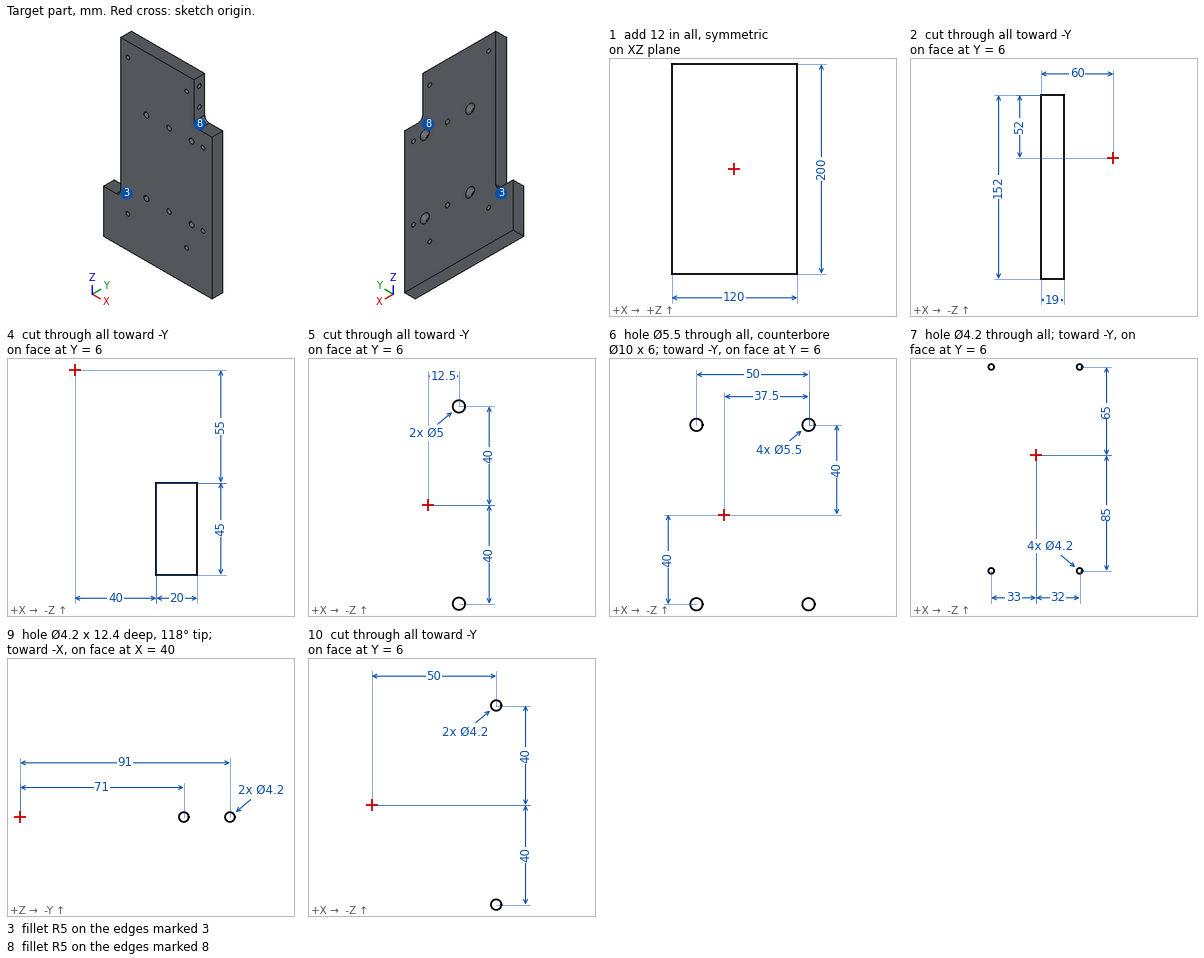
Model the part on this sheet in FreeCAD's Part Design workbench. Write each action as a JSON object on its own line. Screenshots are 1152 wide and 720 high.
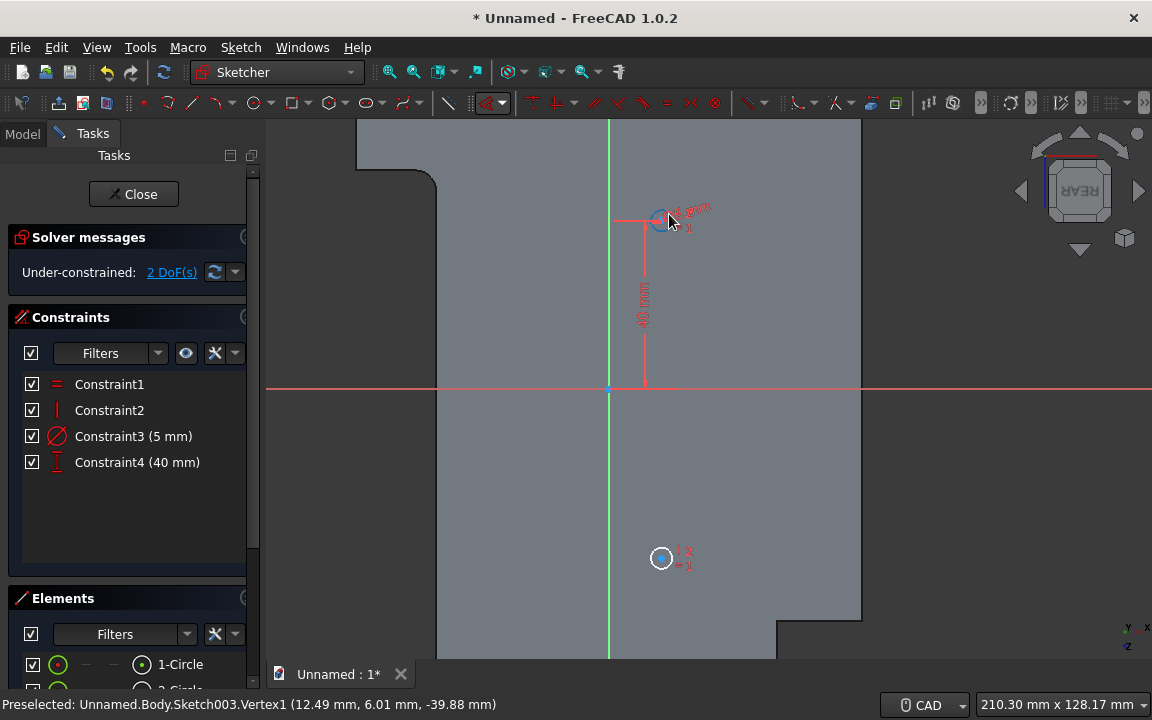
{"action": "left_click", "coordinate": [662, 558]}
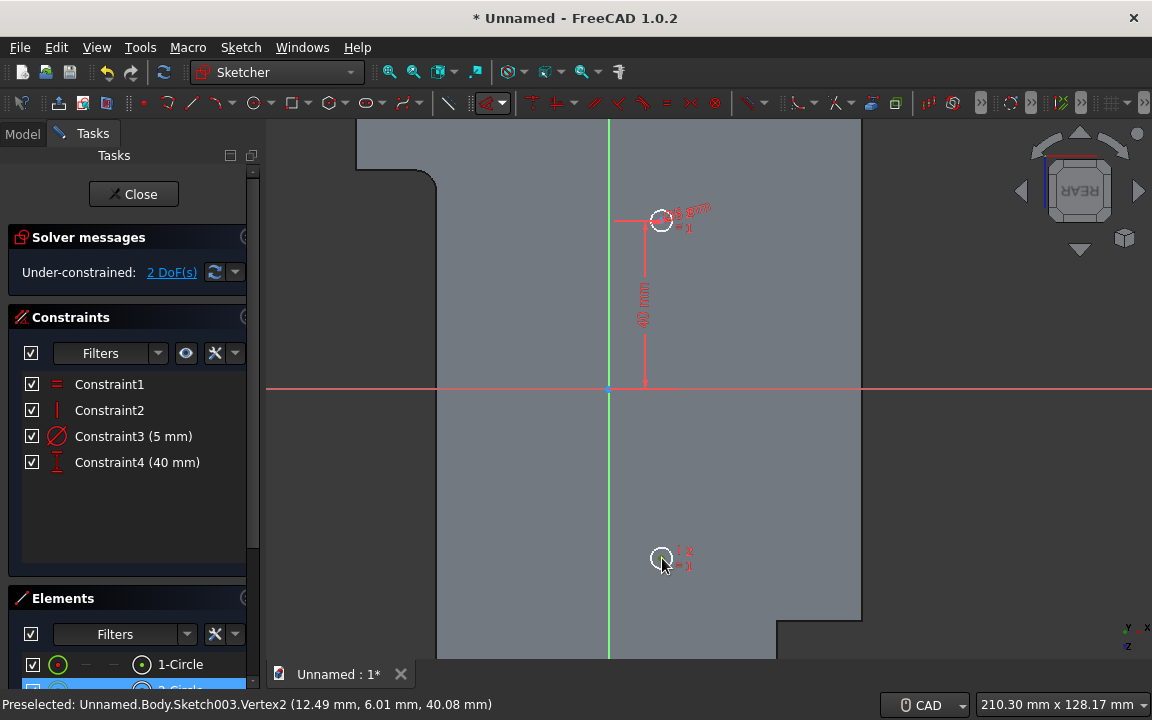
{"action": "left_click", "coordinate": [504, 104]}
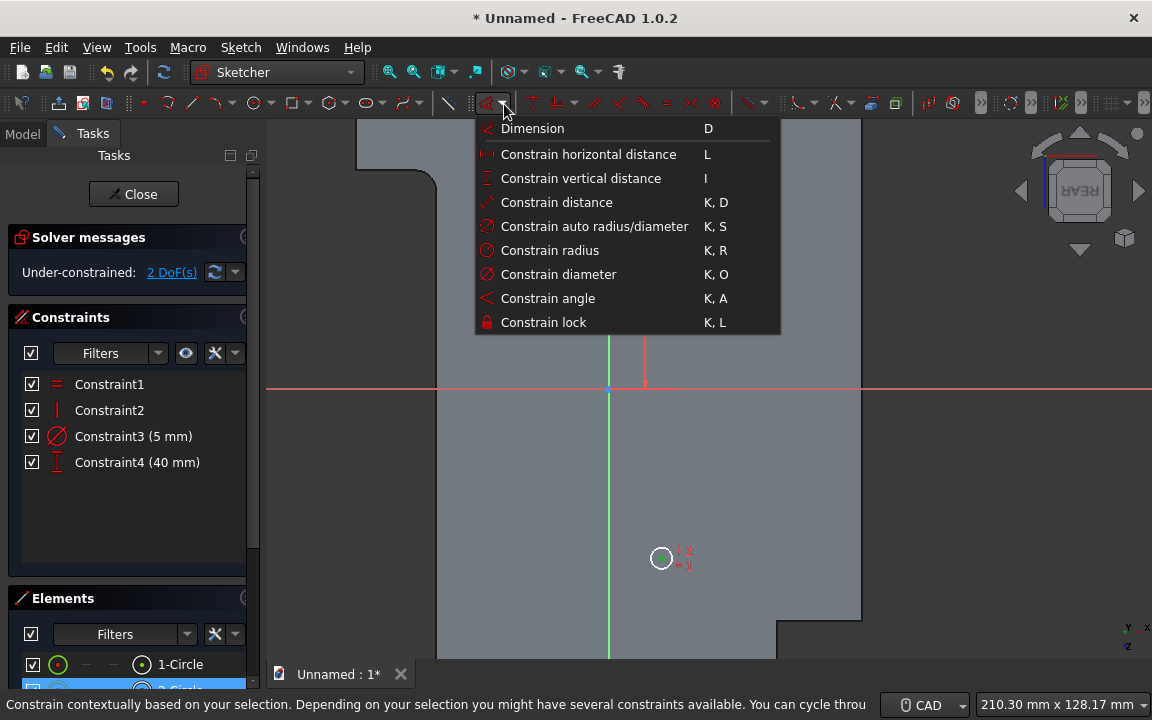
{"action": "left_click", "coordinate": [628, 178]}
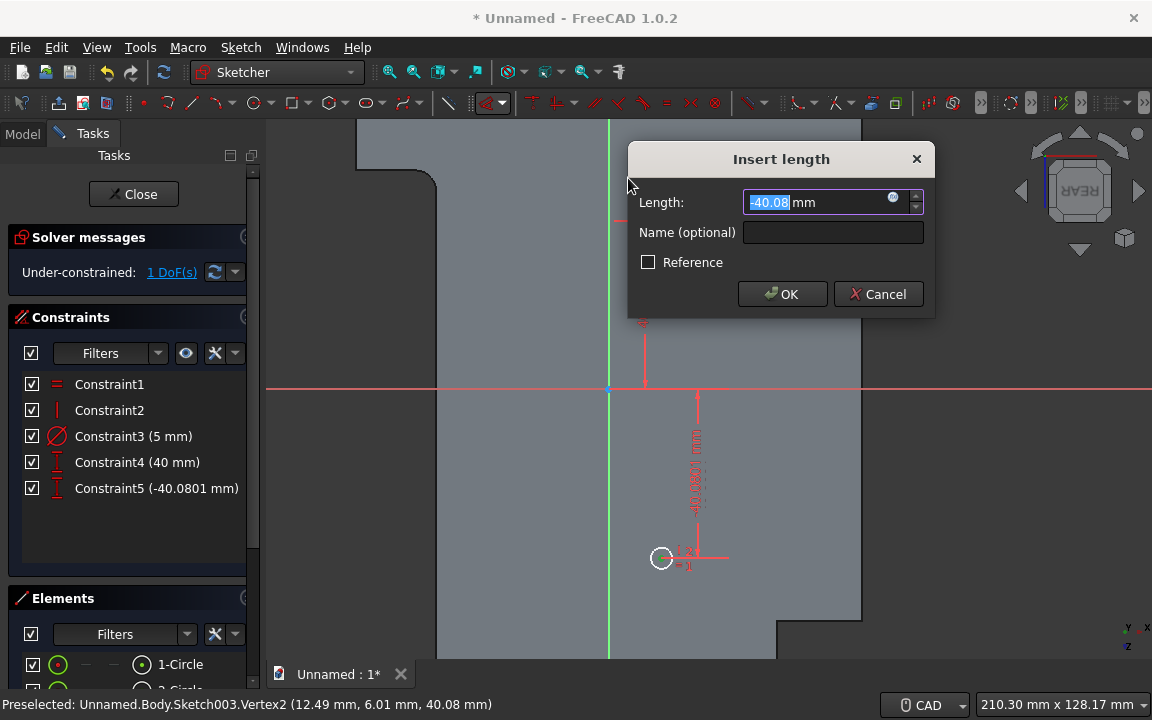
{"action": "type", "text": "-40"}
{"action": "key", "text": "Return"}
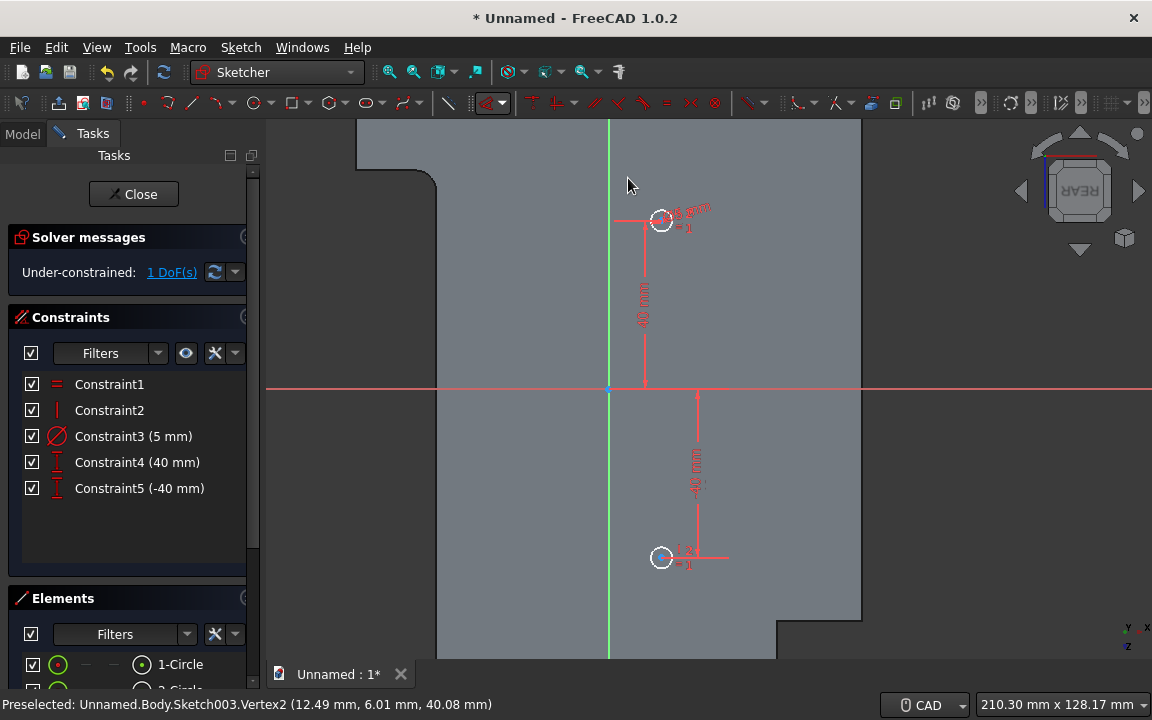
{"action": "left_click", "coordinate": [662, 221]}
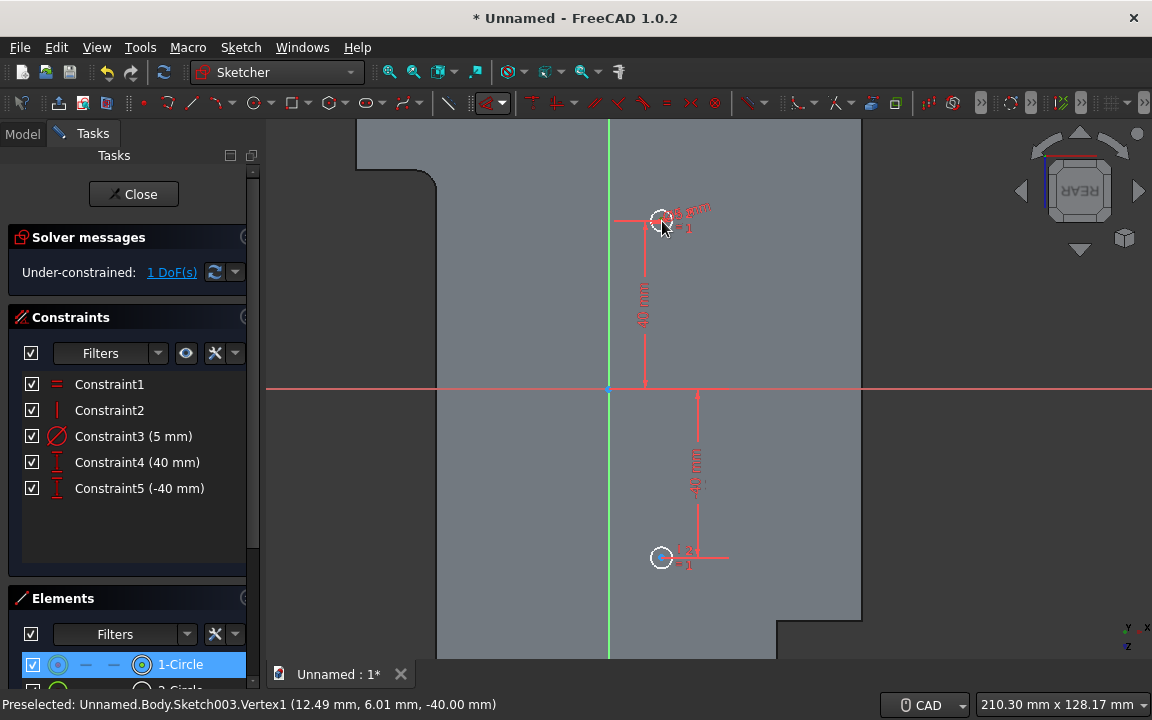
{"action": "key", "text": "l"}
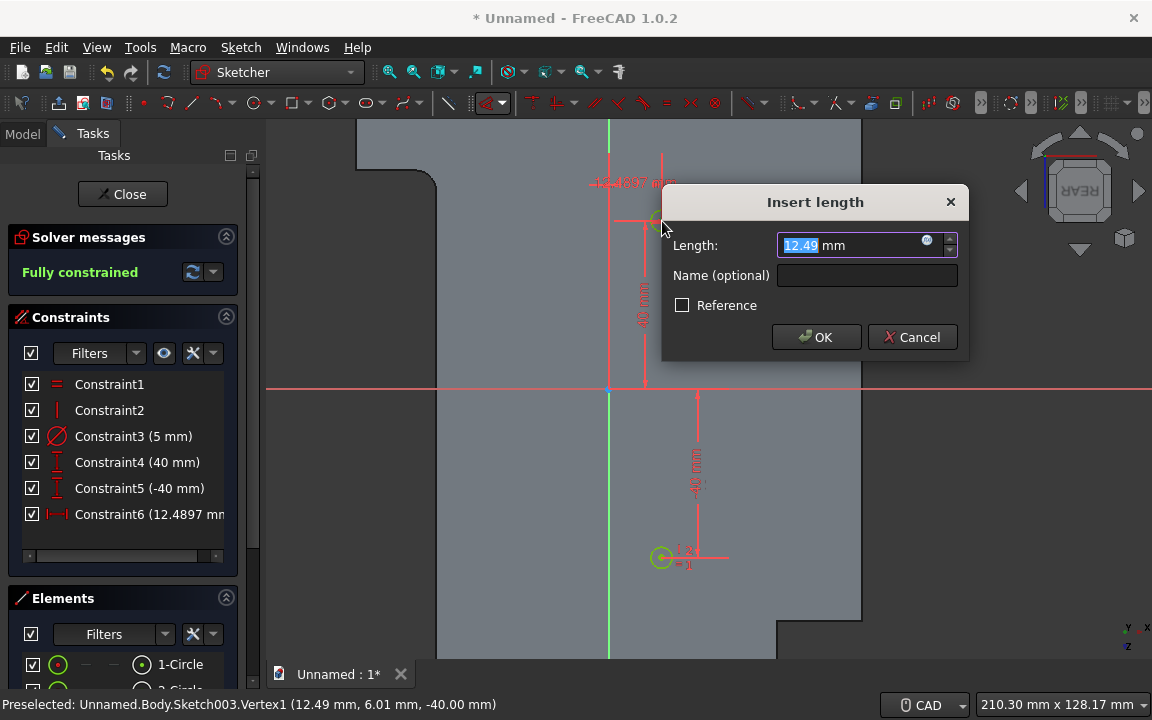
{"action": "type", "text": "12.5"}
{"action": "key", "text": "Return"}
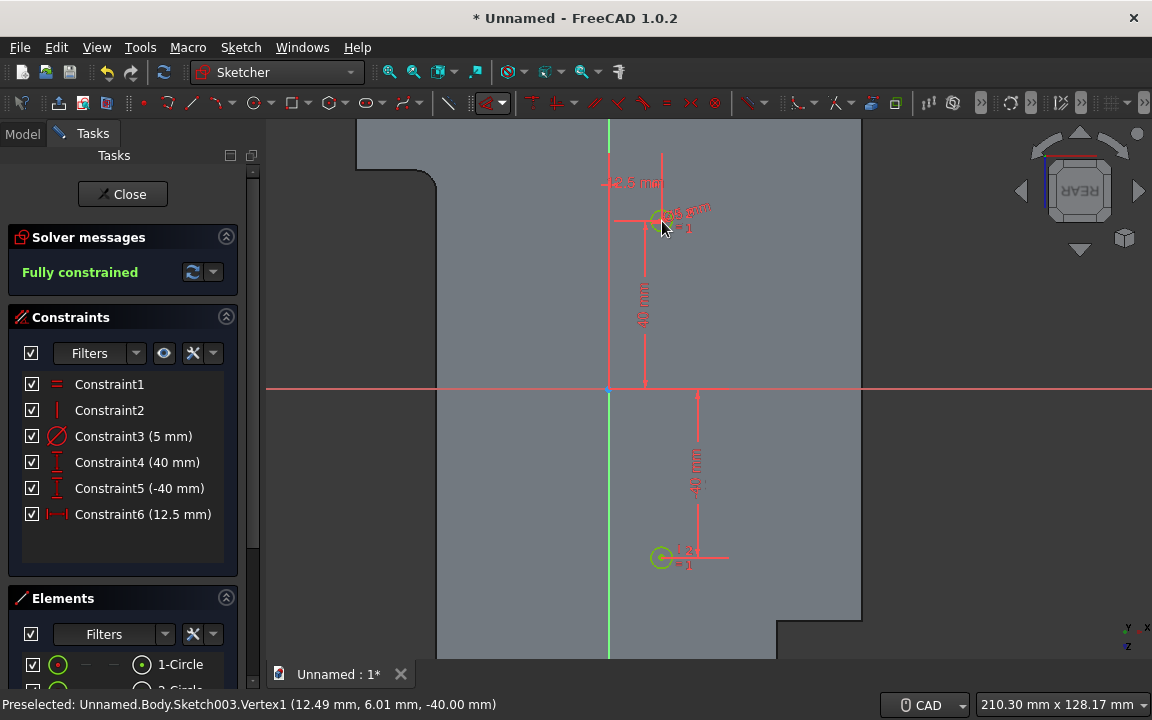
{"action": "left_click", "coordinate": [123, 194]}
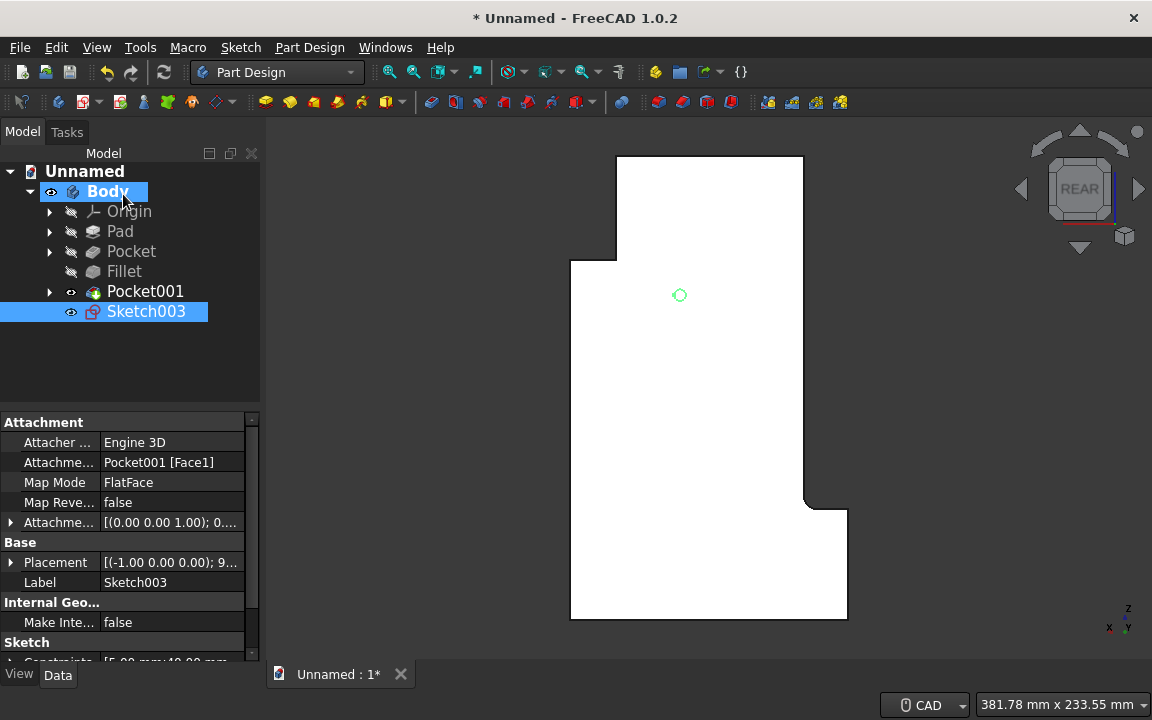
{"action": "left_click", "coordinate": [432, 102]}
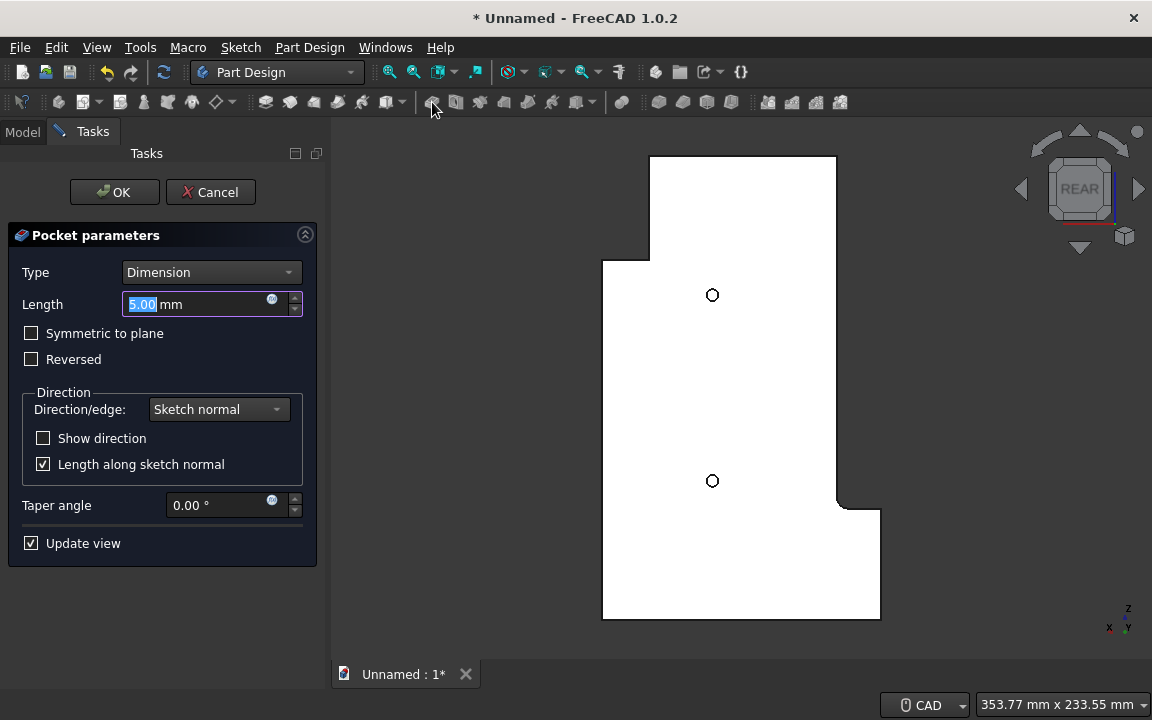
{"action": "left_click", "coordinate": [212, 272]}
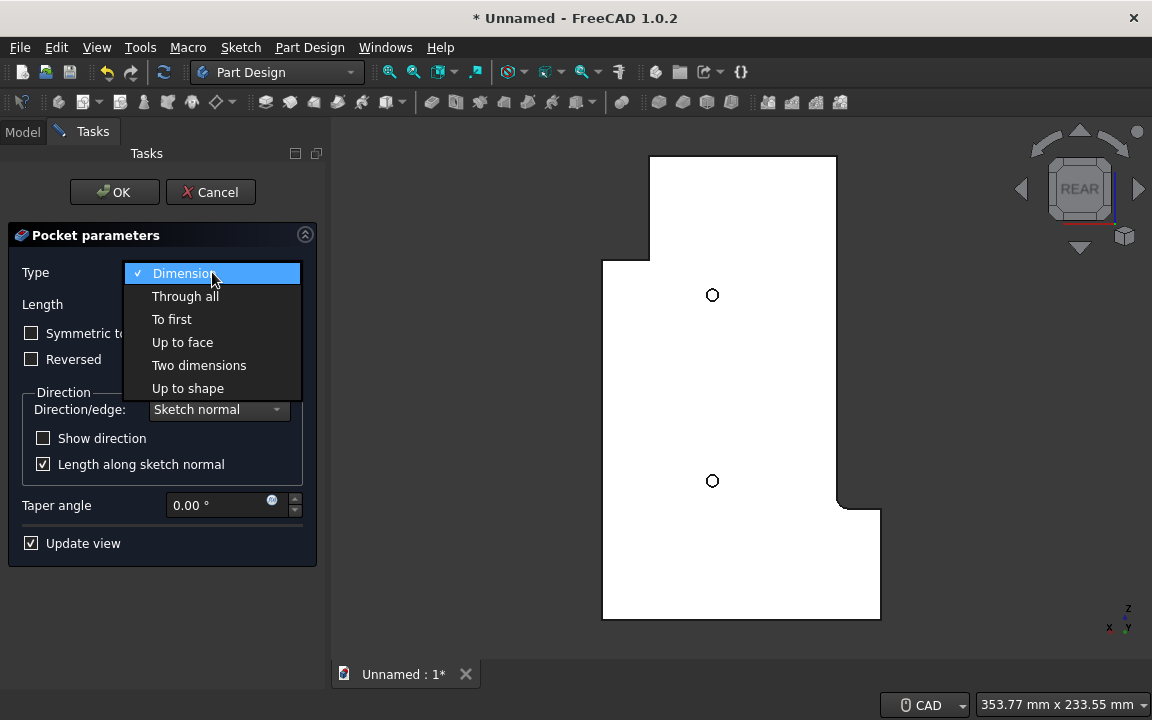
{"action": "left_click", "coordinate": [212, 296]}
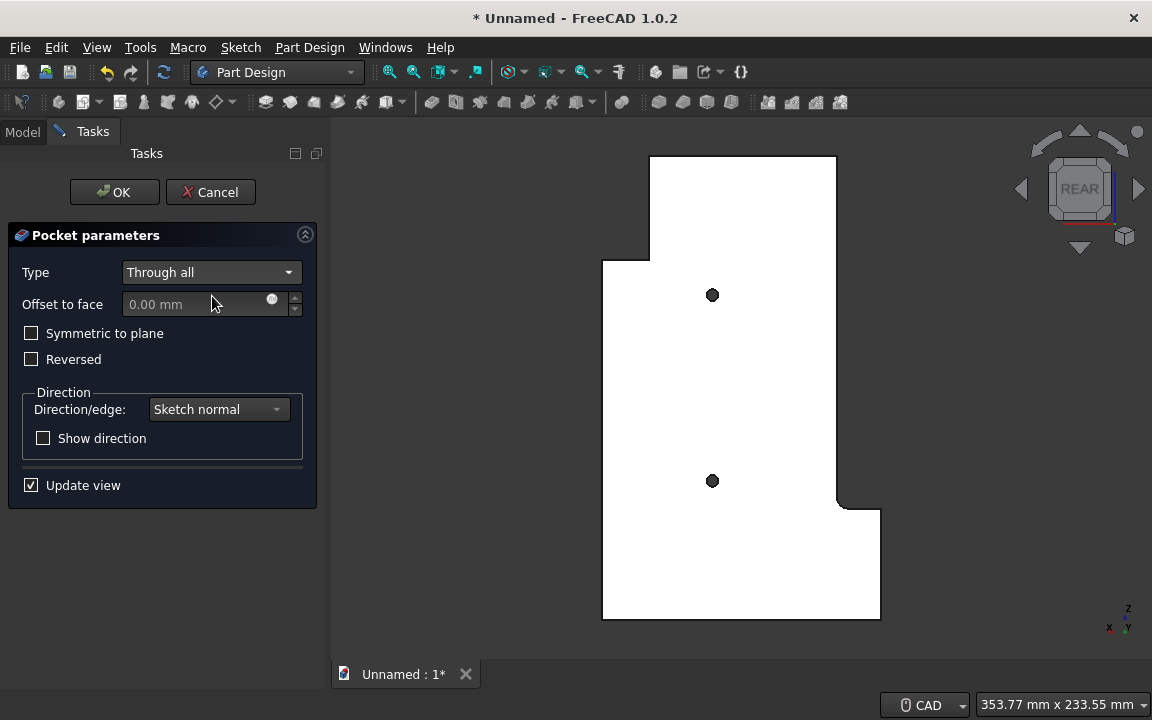
{"action": "left_click", "coordinate": [115, 192]}